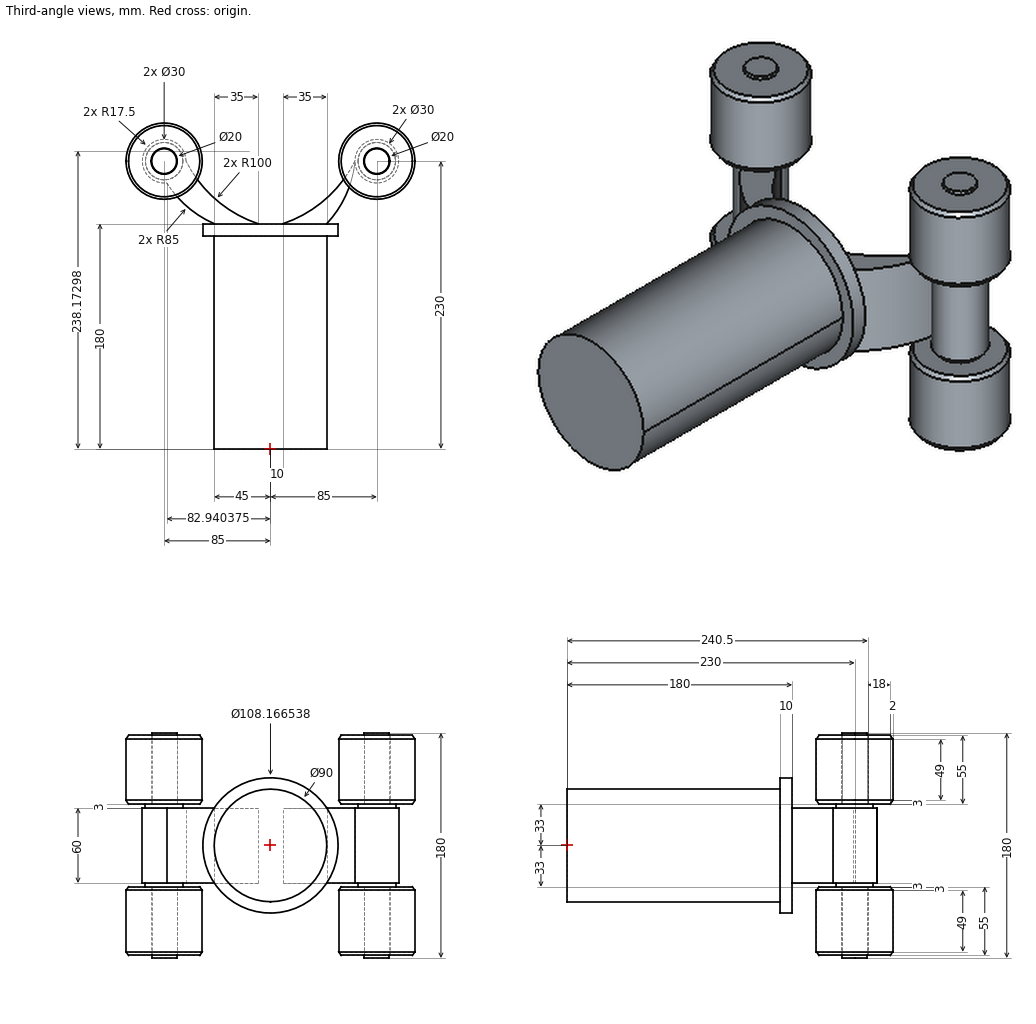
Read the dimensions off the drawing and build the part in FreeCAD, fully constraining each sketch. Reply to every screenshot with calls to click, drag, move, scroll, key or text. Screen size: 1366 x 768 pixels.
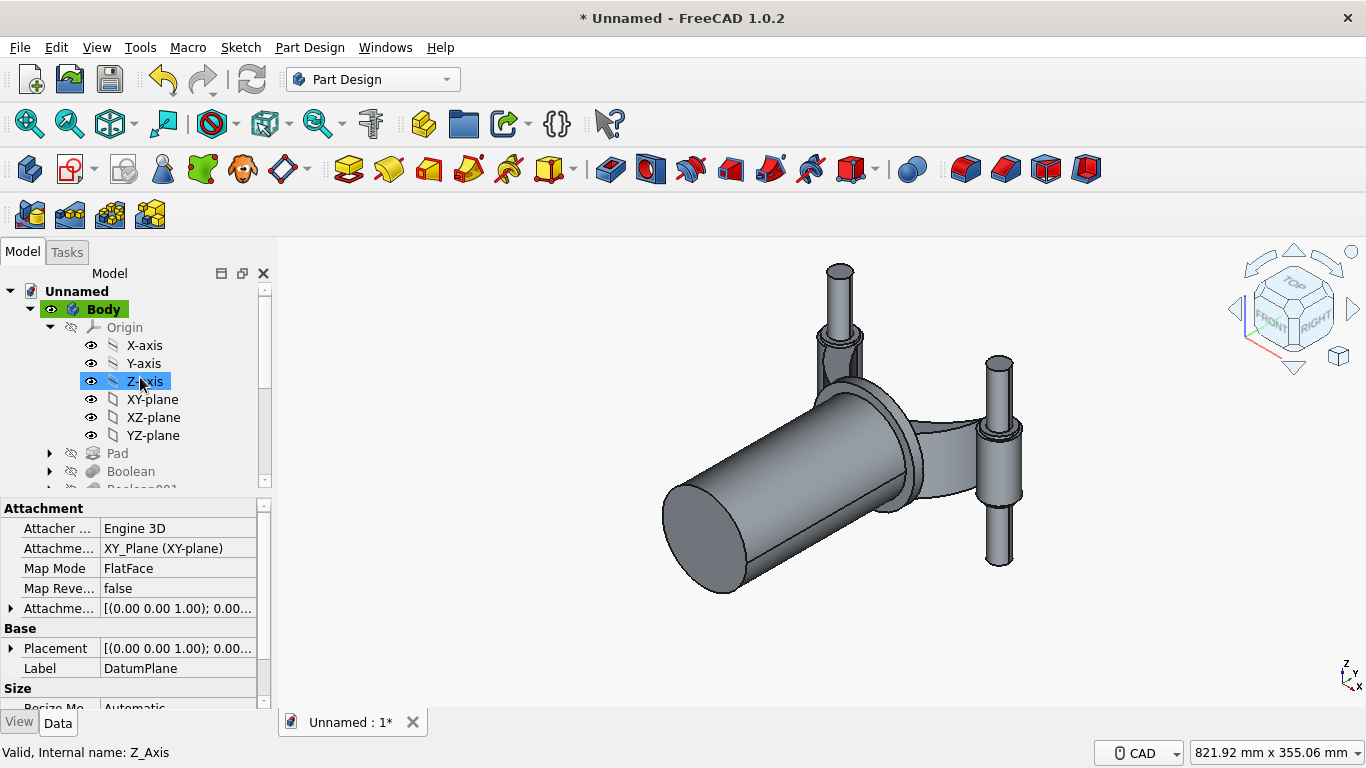
click(136, 435)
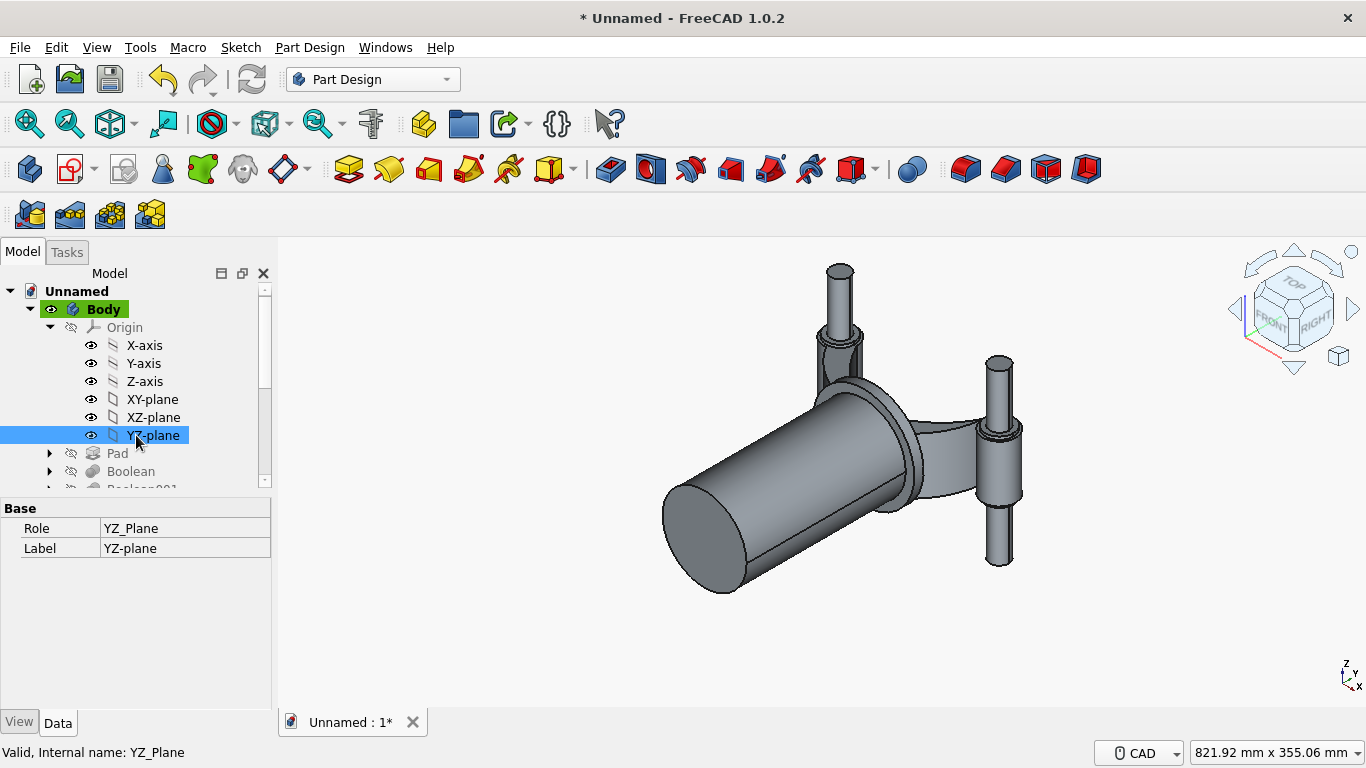
click(284, 170)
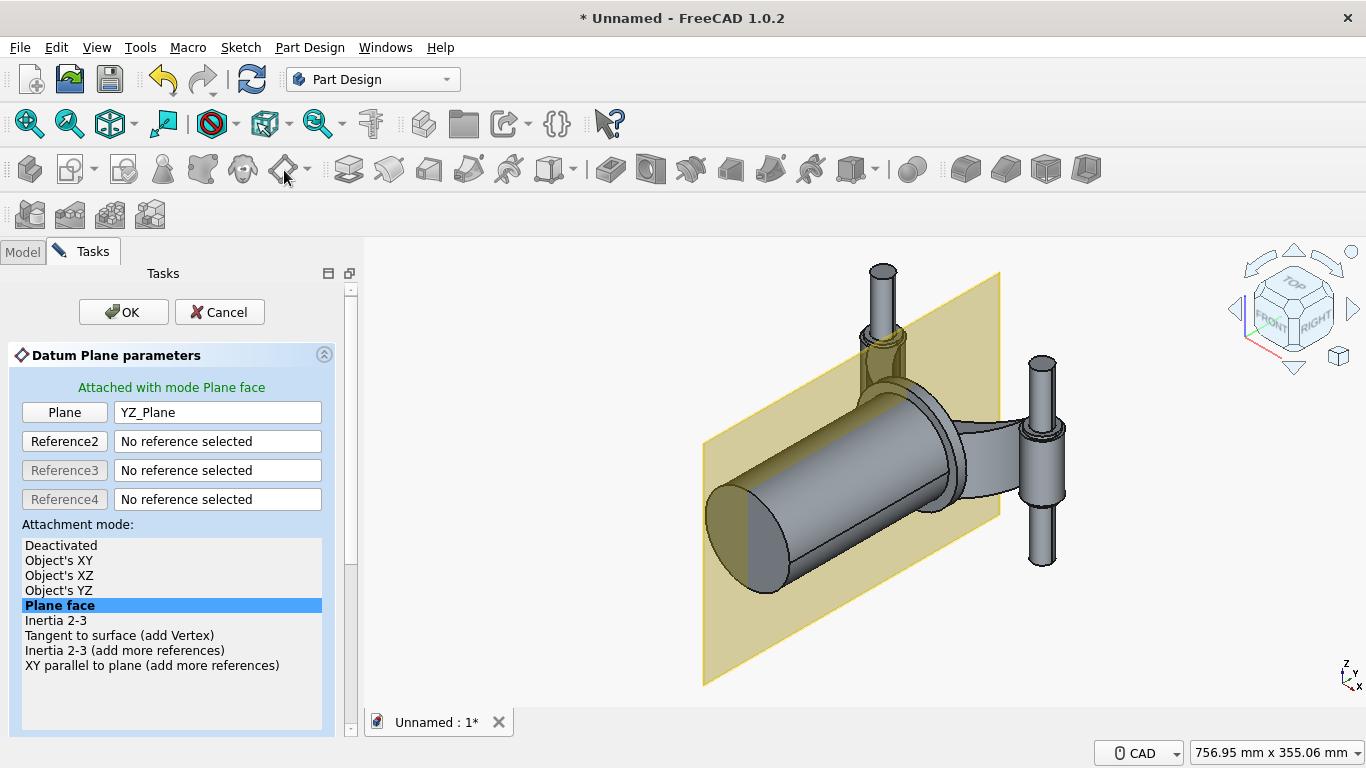
scroll(351, 510, down, 3)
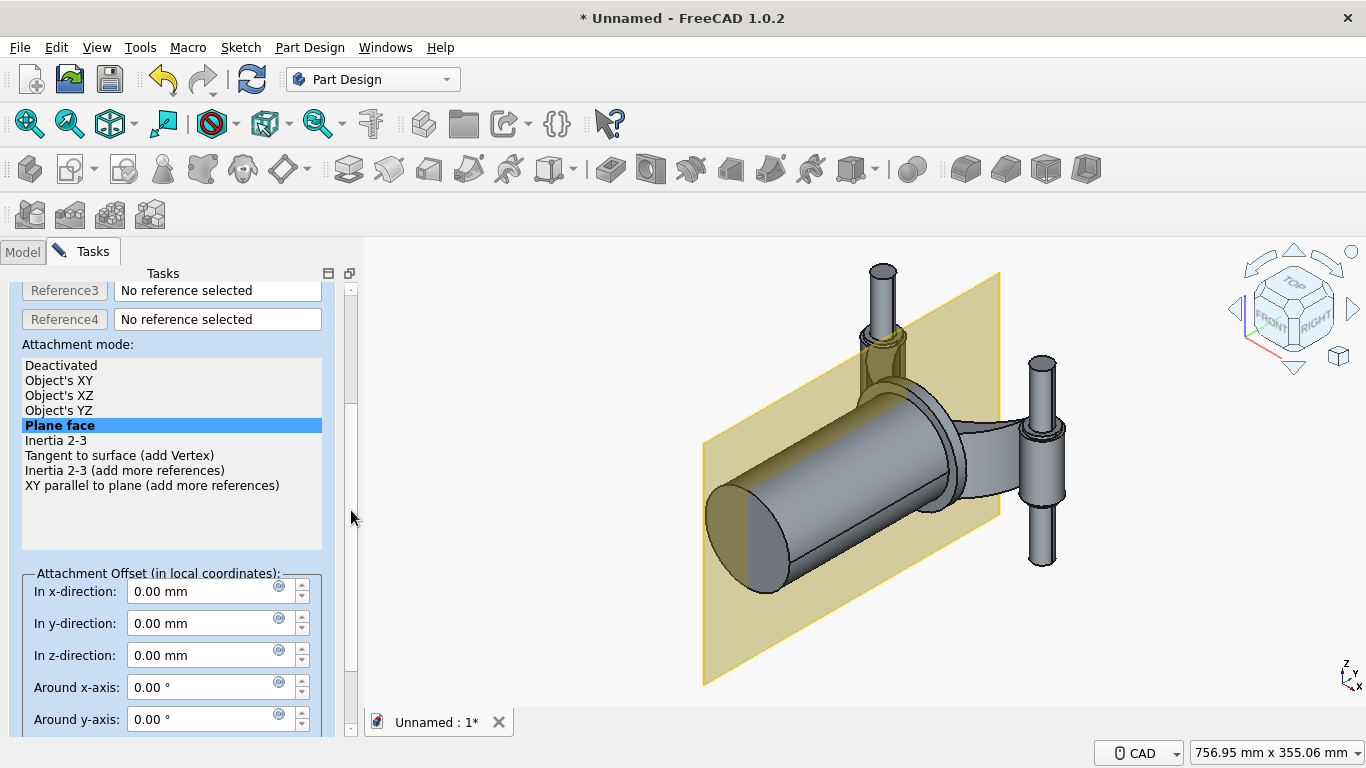
triple_click(210, 655)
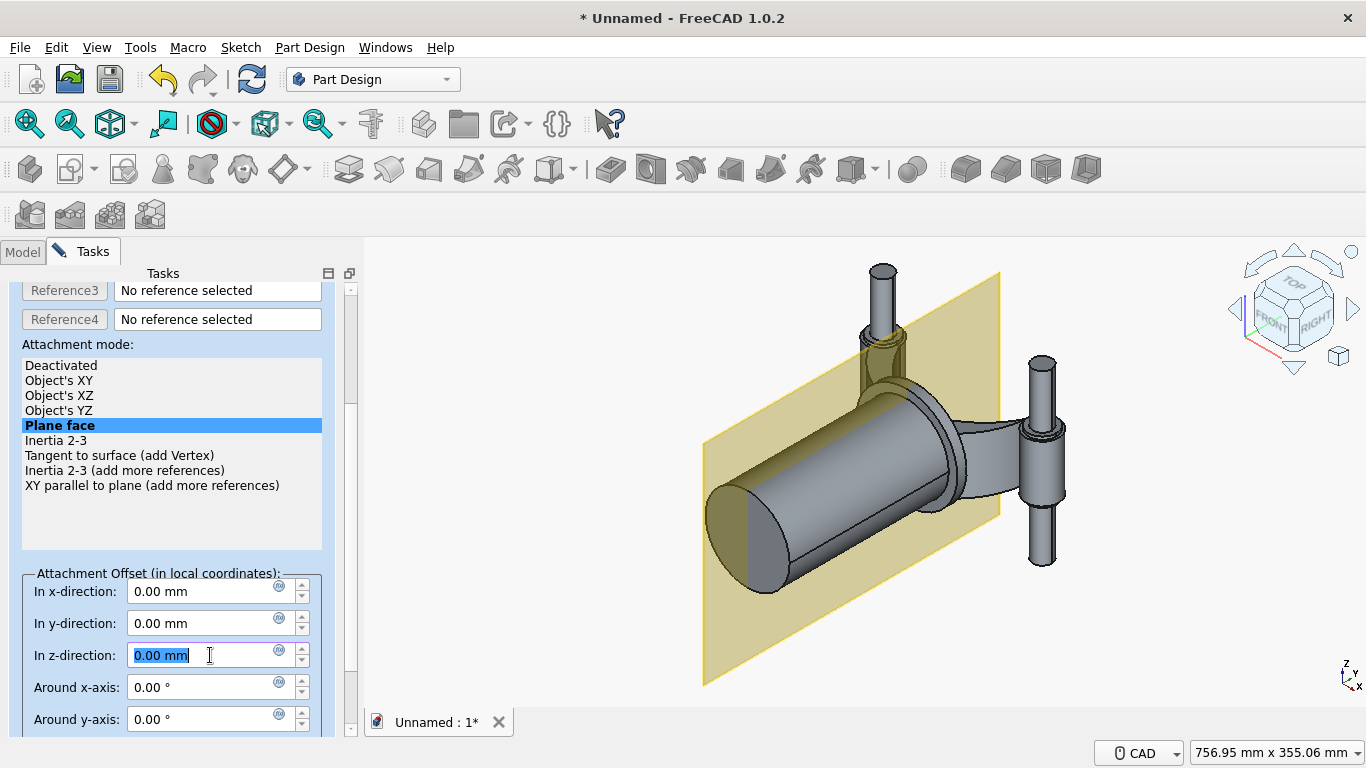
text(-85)
key(Tab)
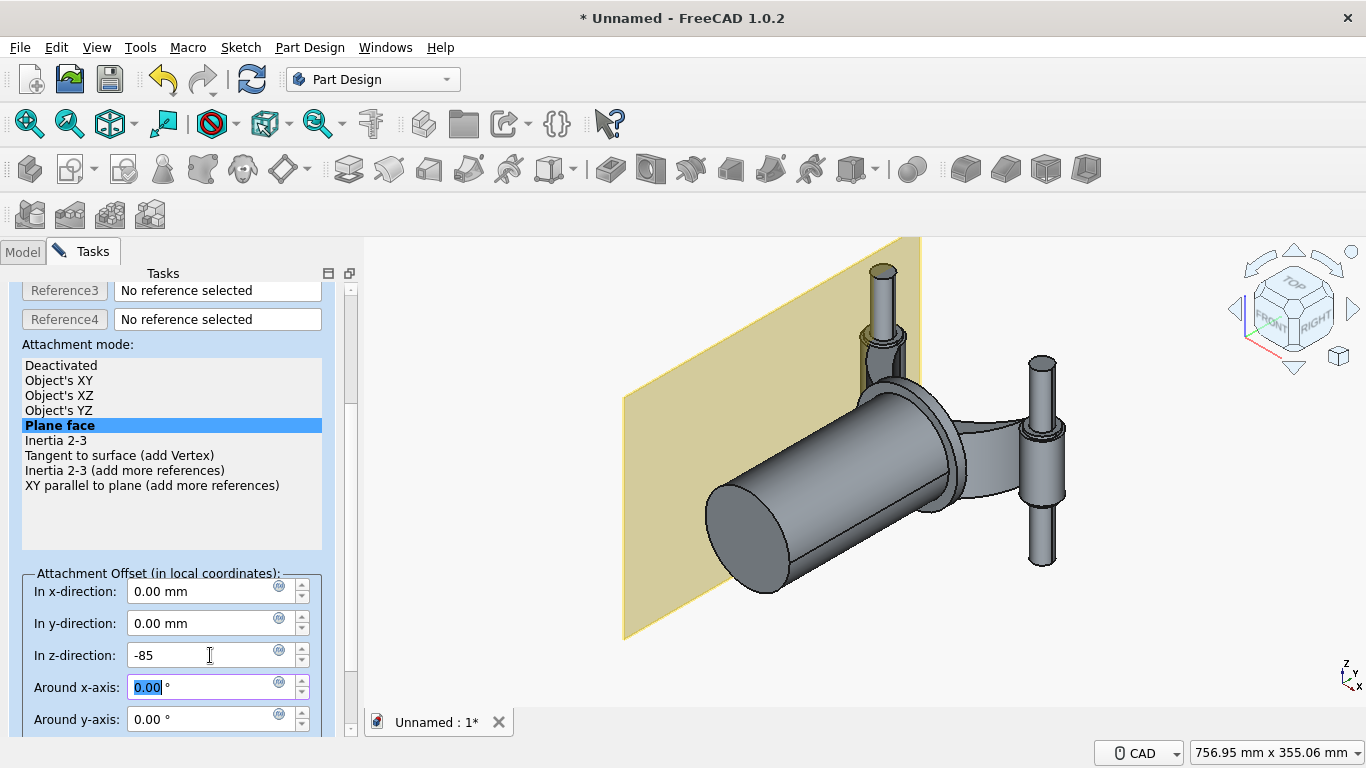
scroll(351, 510, up, 4)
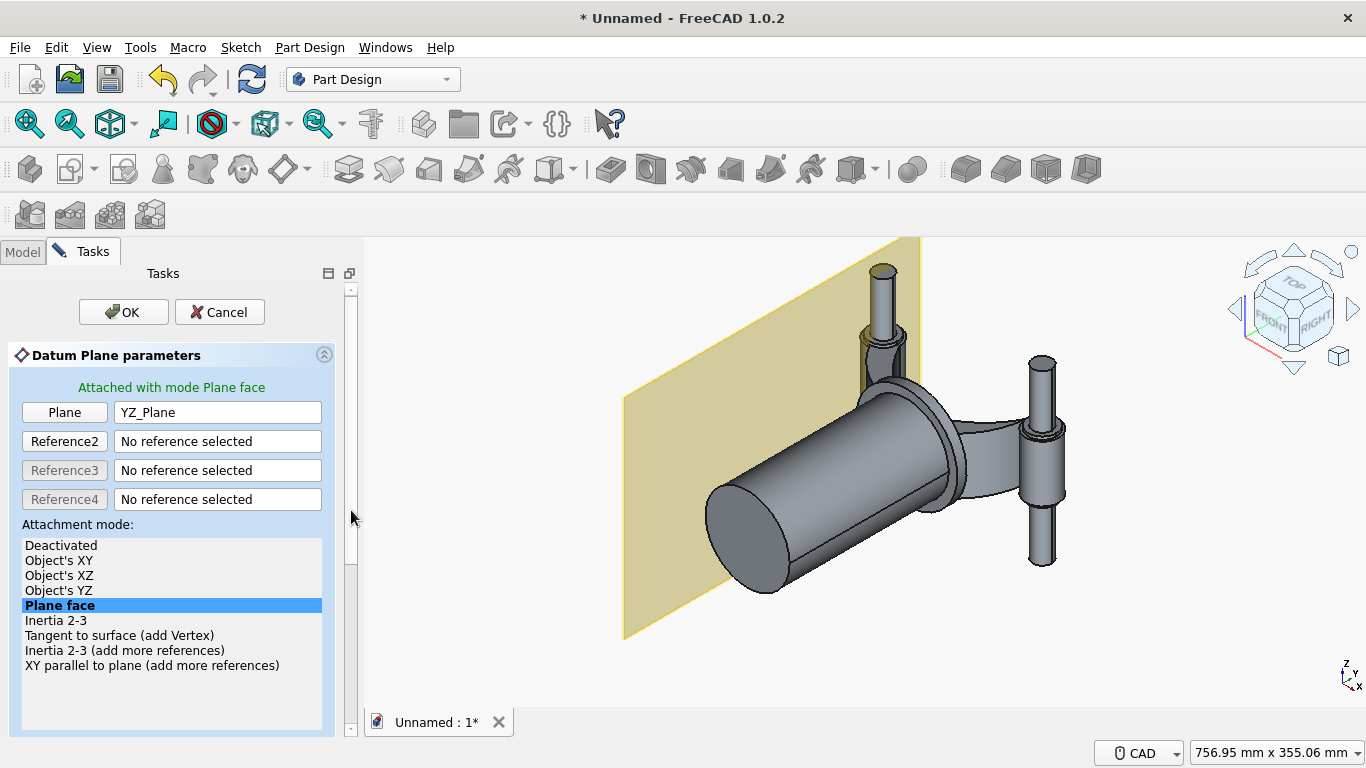
click(124, 312)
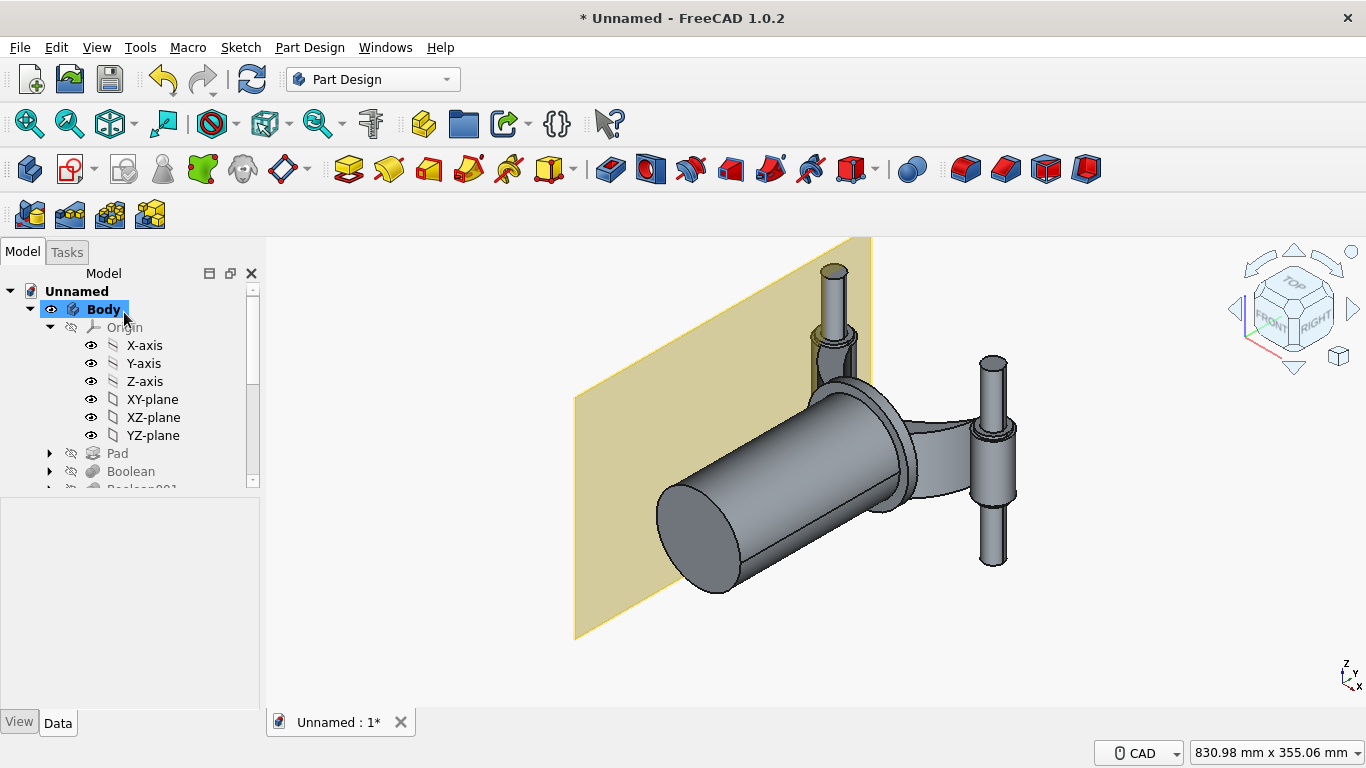
scroll(100, 377, down, 3)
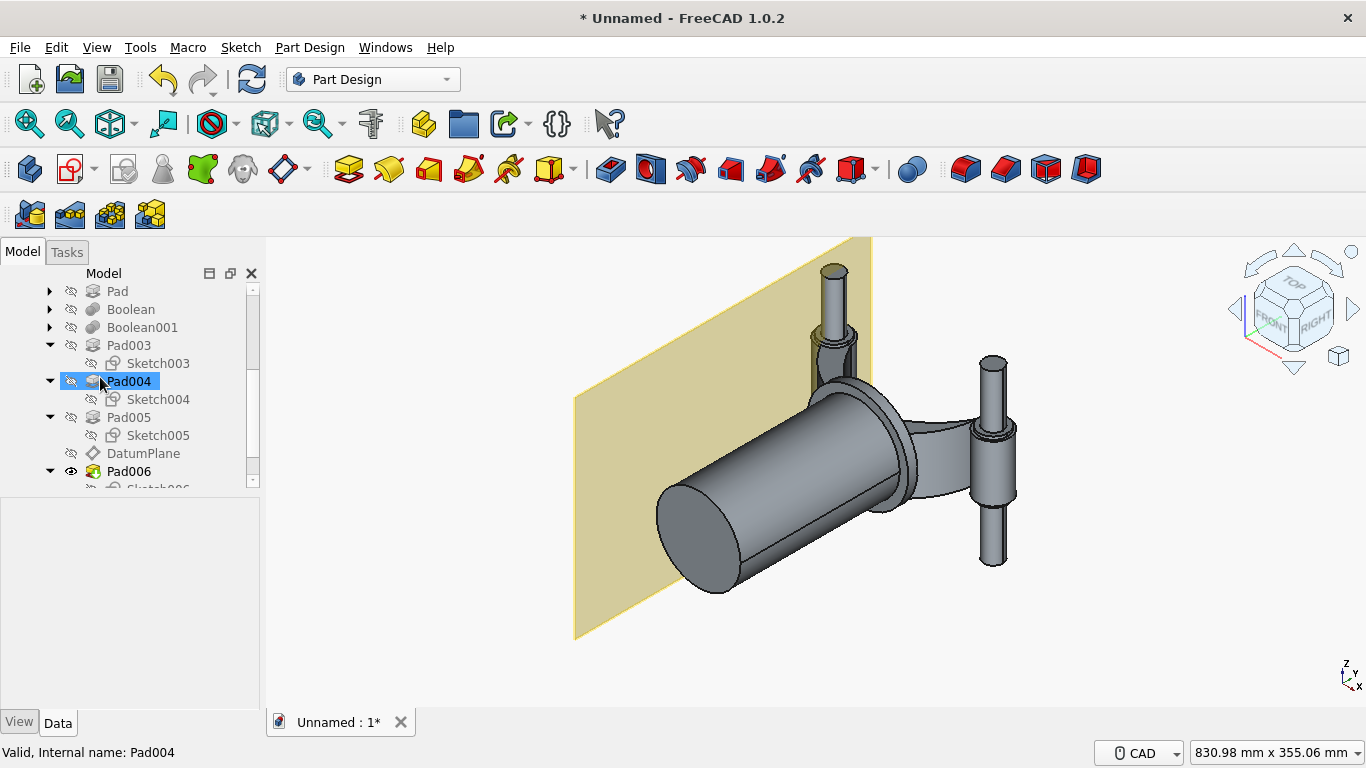
scroll(140, 377, up, 15)